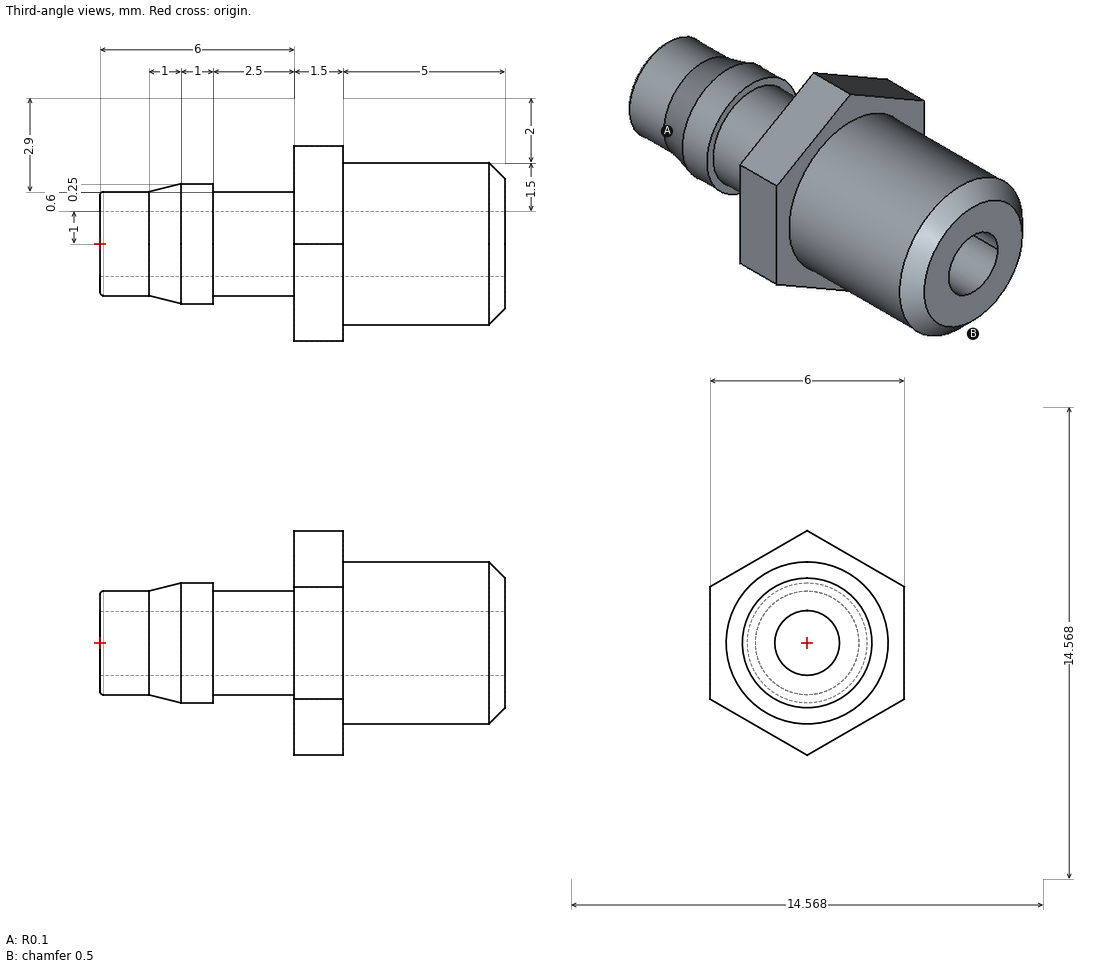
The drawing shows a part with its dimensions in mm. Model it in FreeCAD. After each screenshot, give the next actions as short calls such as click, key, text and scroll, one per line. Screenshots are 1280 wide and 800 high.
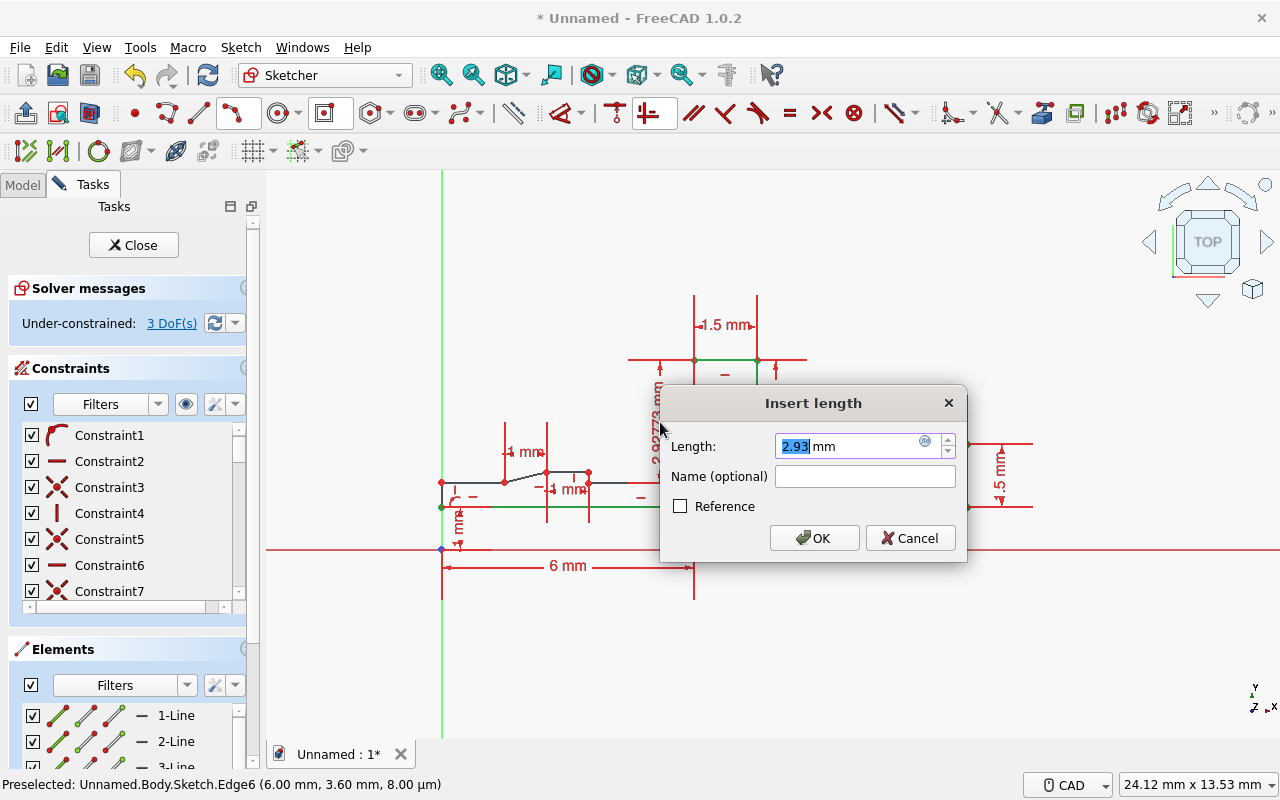
text(2.9)
key(Return)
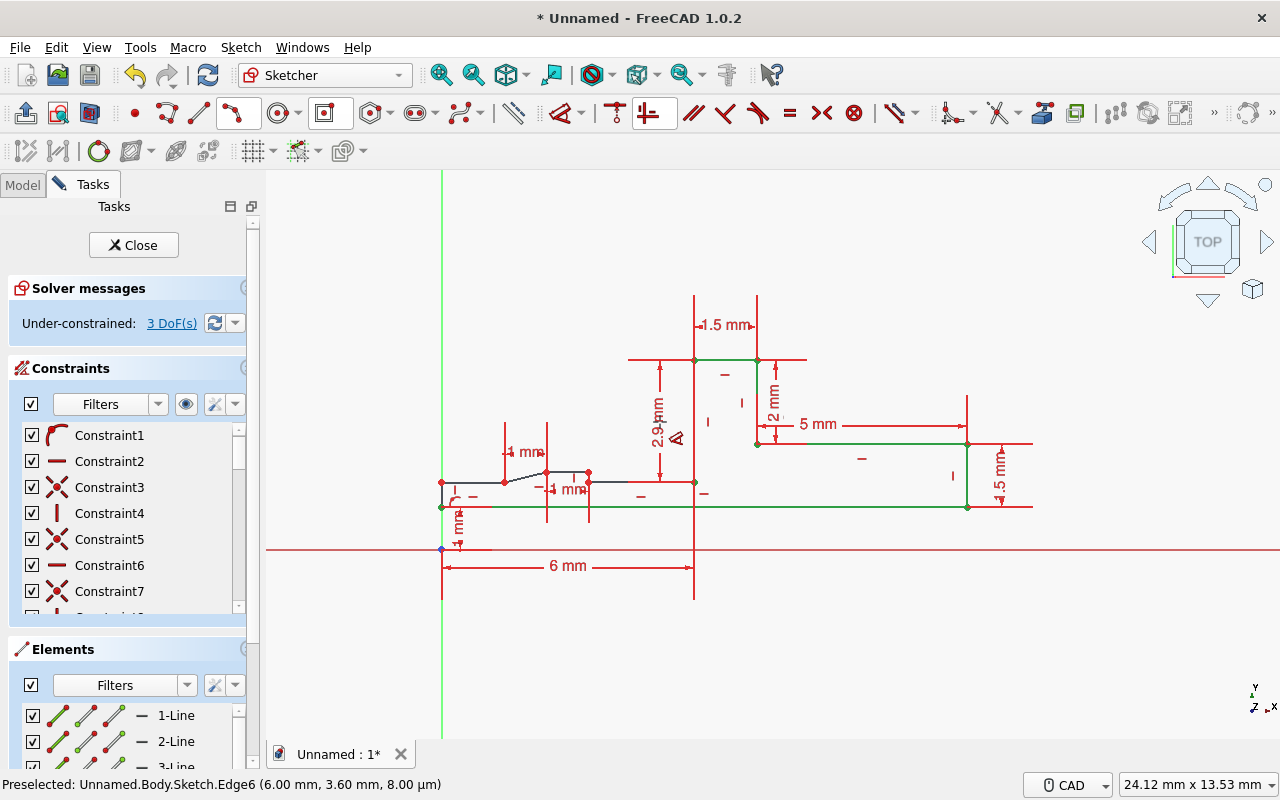
click(662, 482)
click(641, 448)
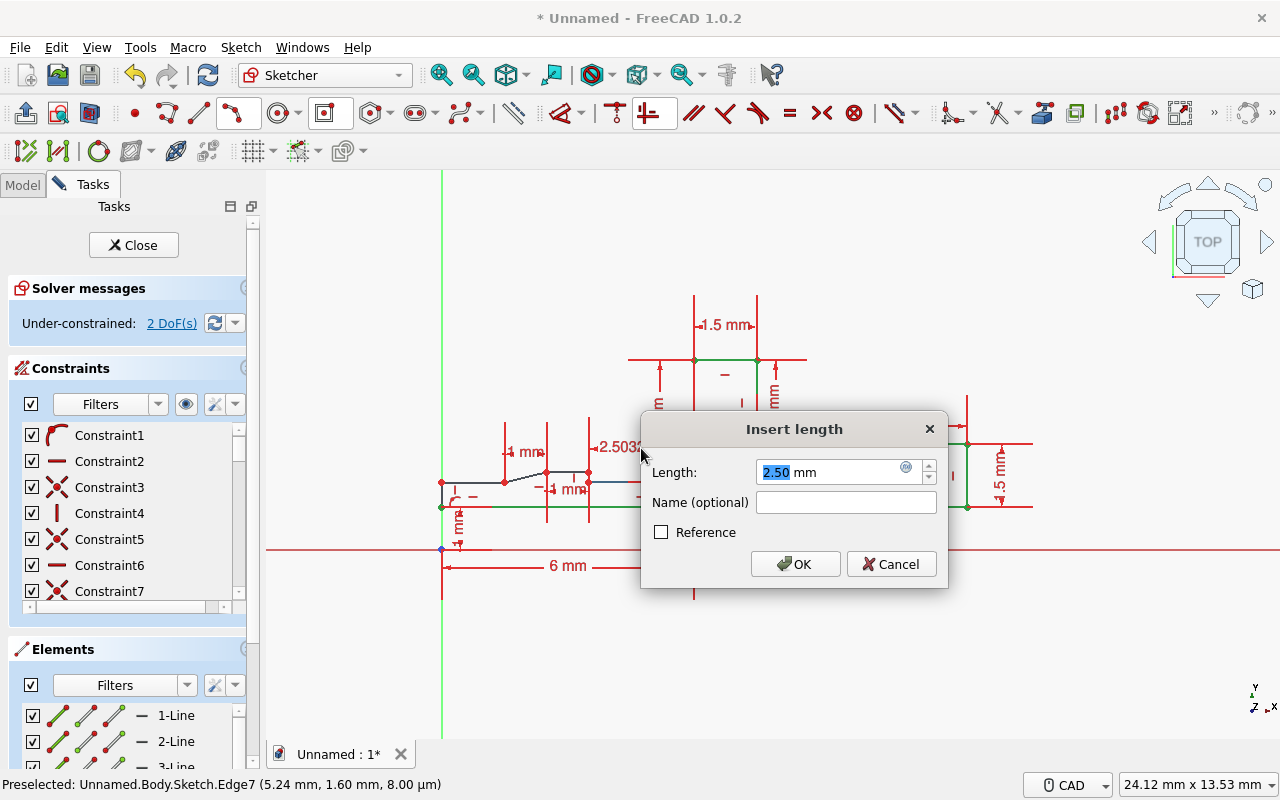
text(2.5)
key(Return)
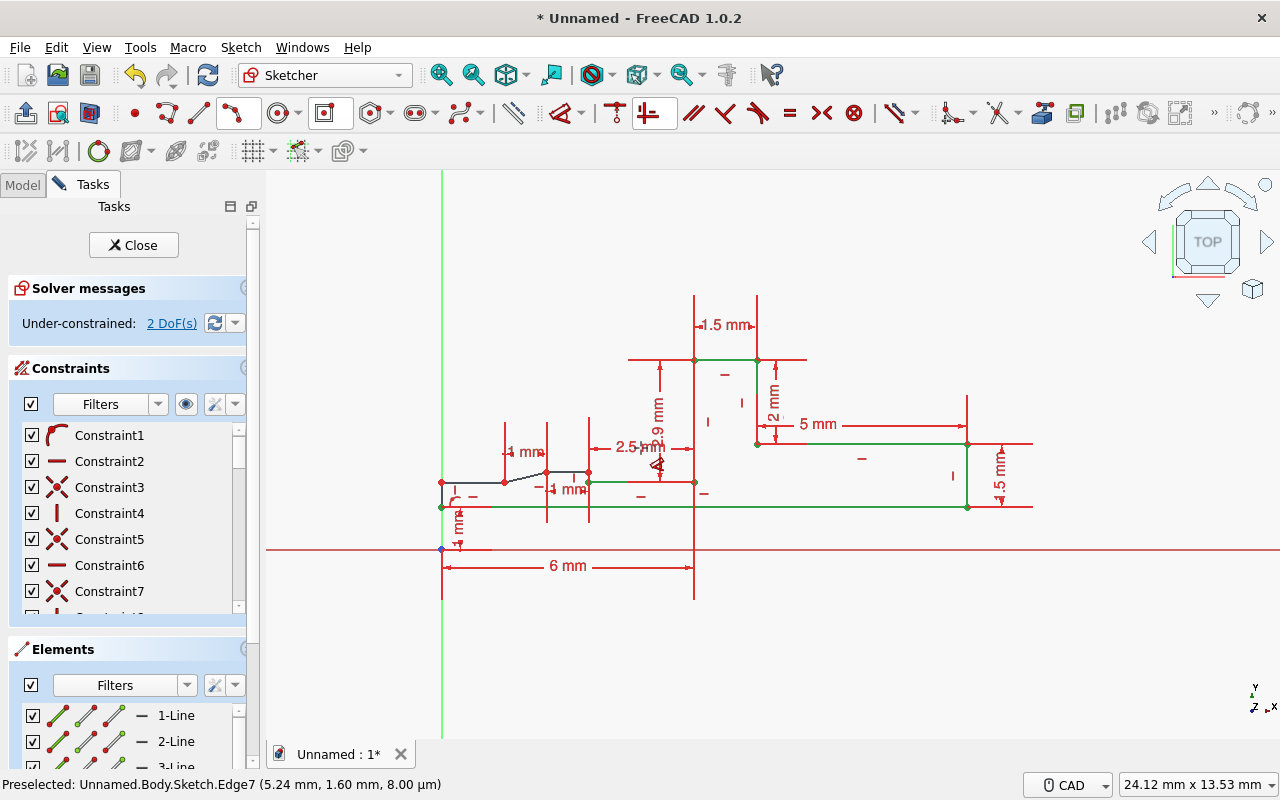
scroll(442, 493, up, 3)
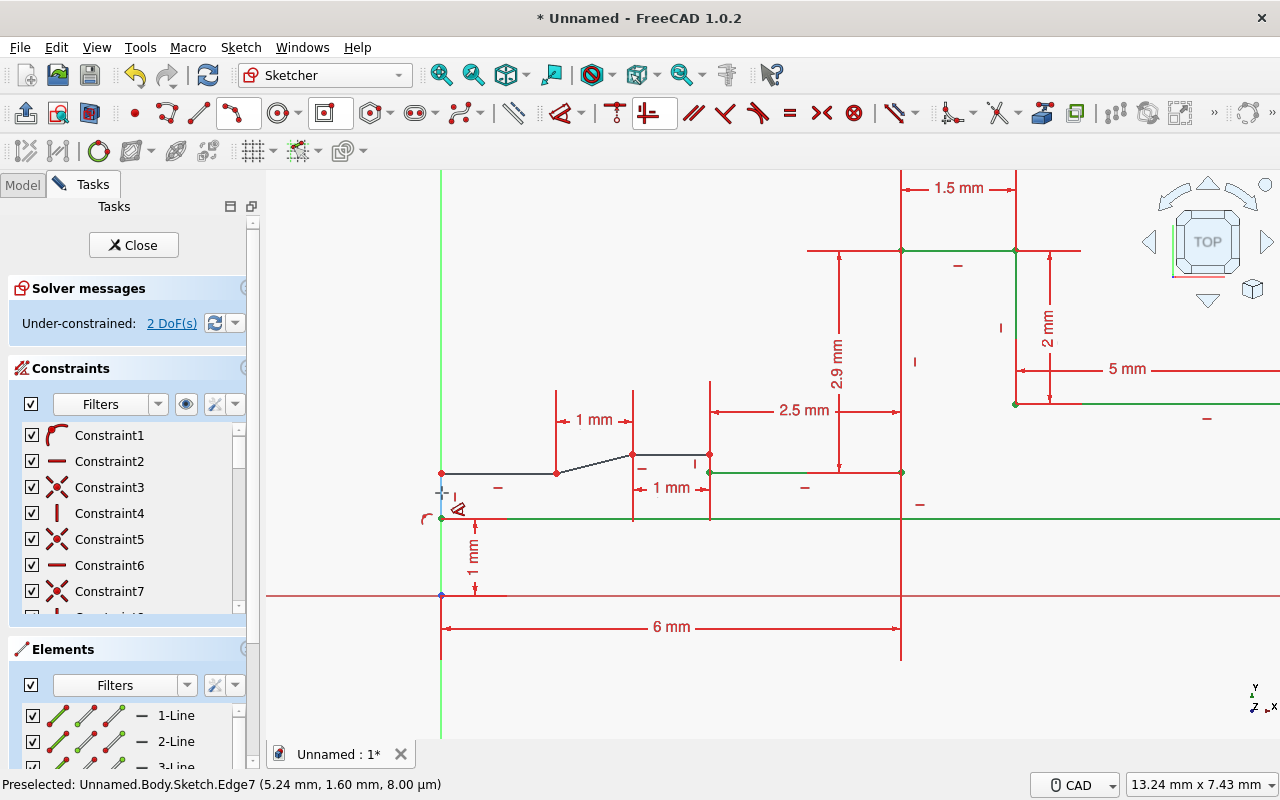
click(441, 492)
click(407, 496)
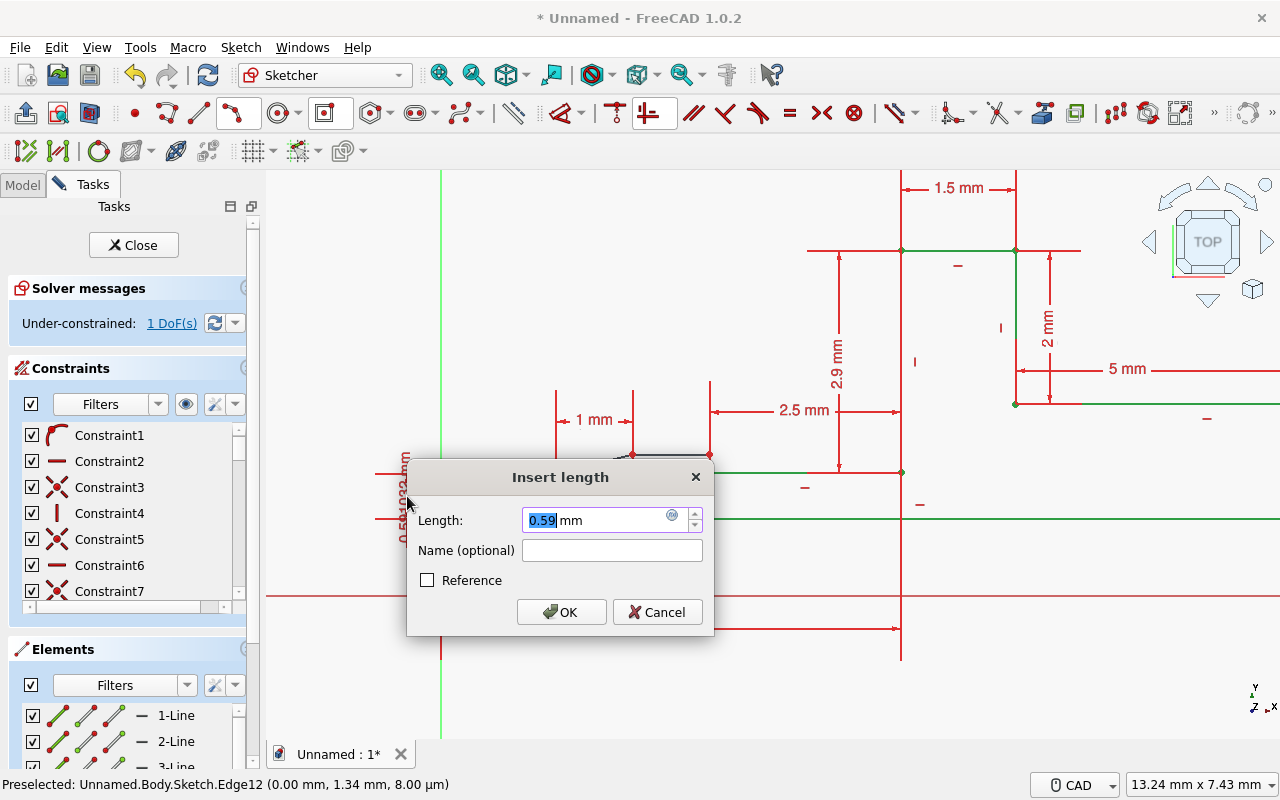
text(0.6)
key(Return)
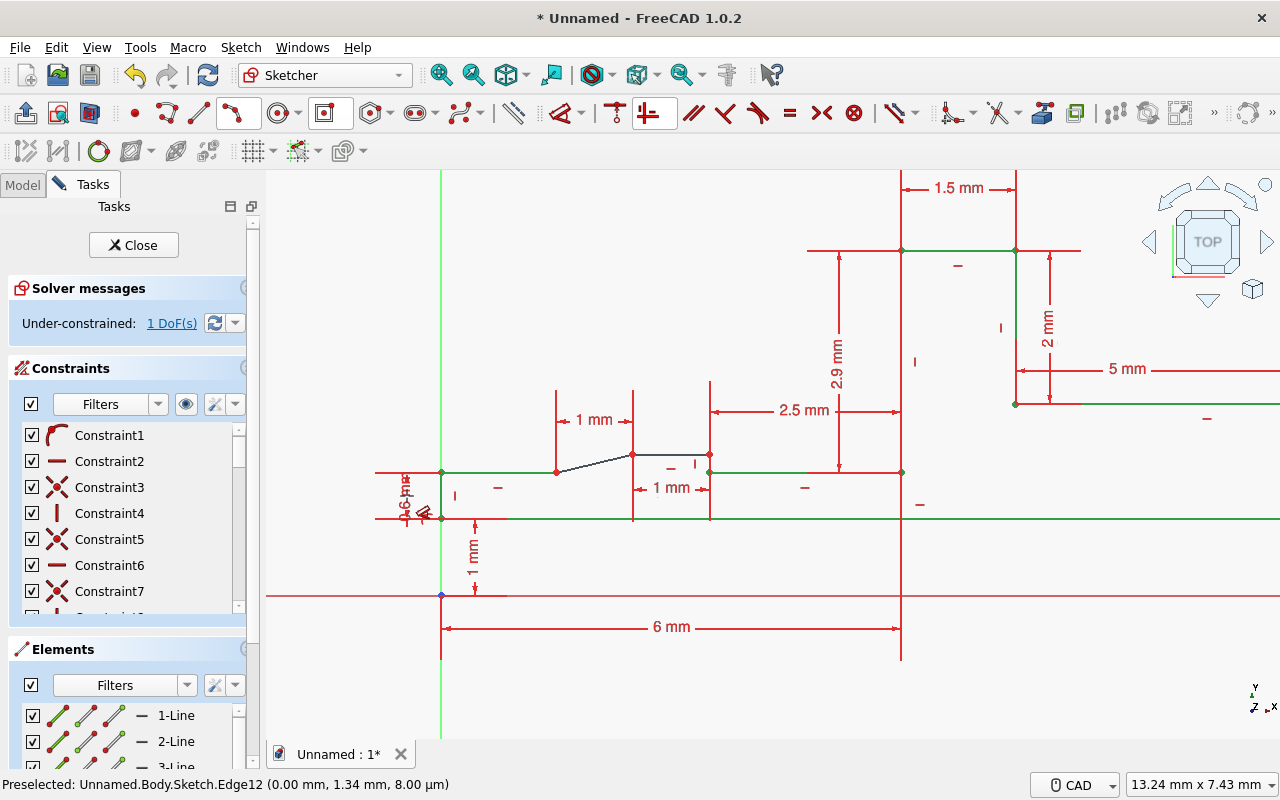
scroll(710, 464, up, 4)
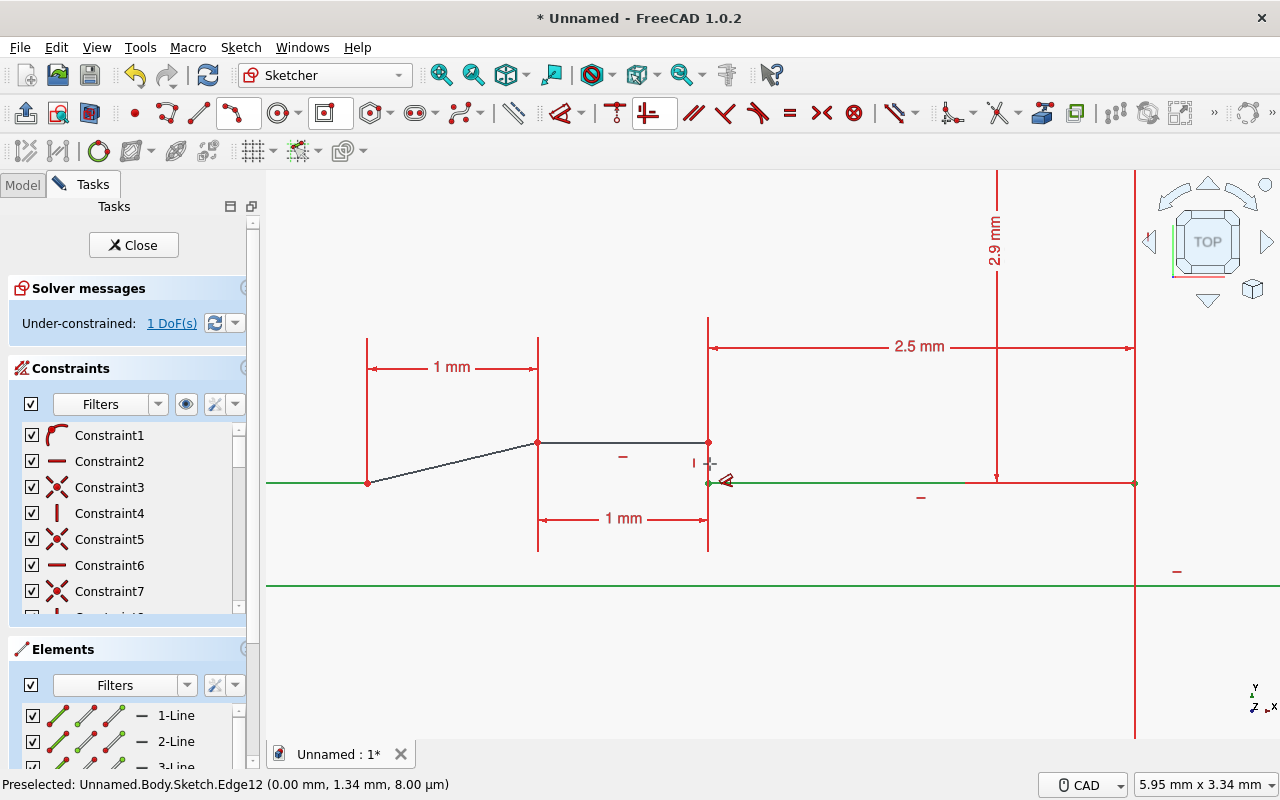
click(708, 463)
click(674, 463)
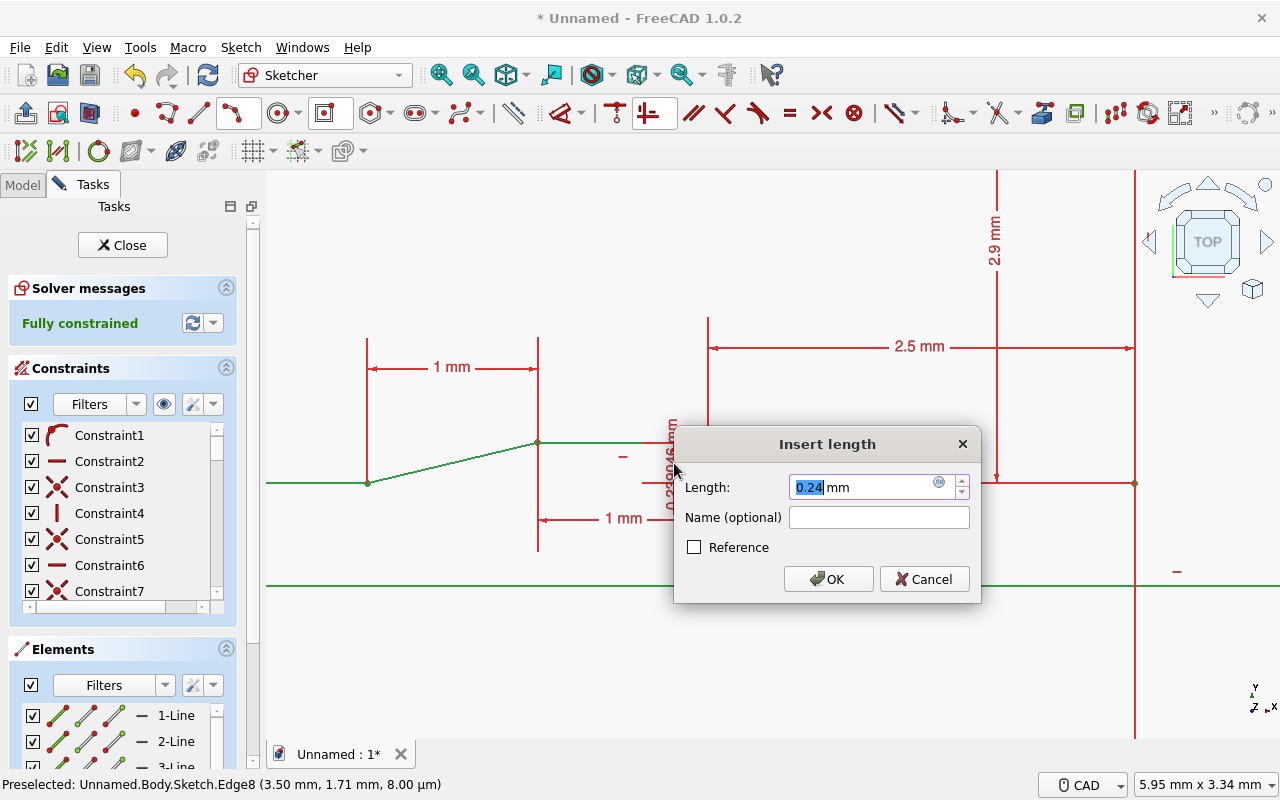
text(0.25)
key(Return)
key(Escape)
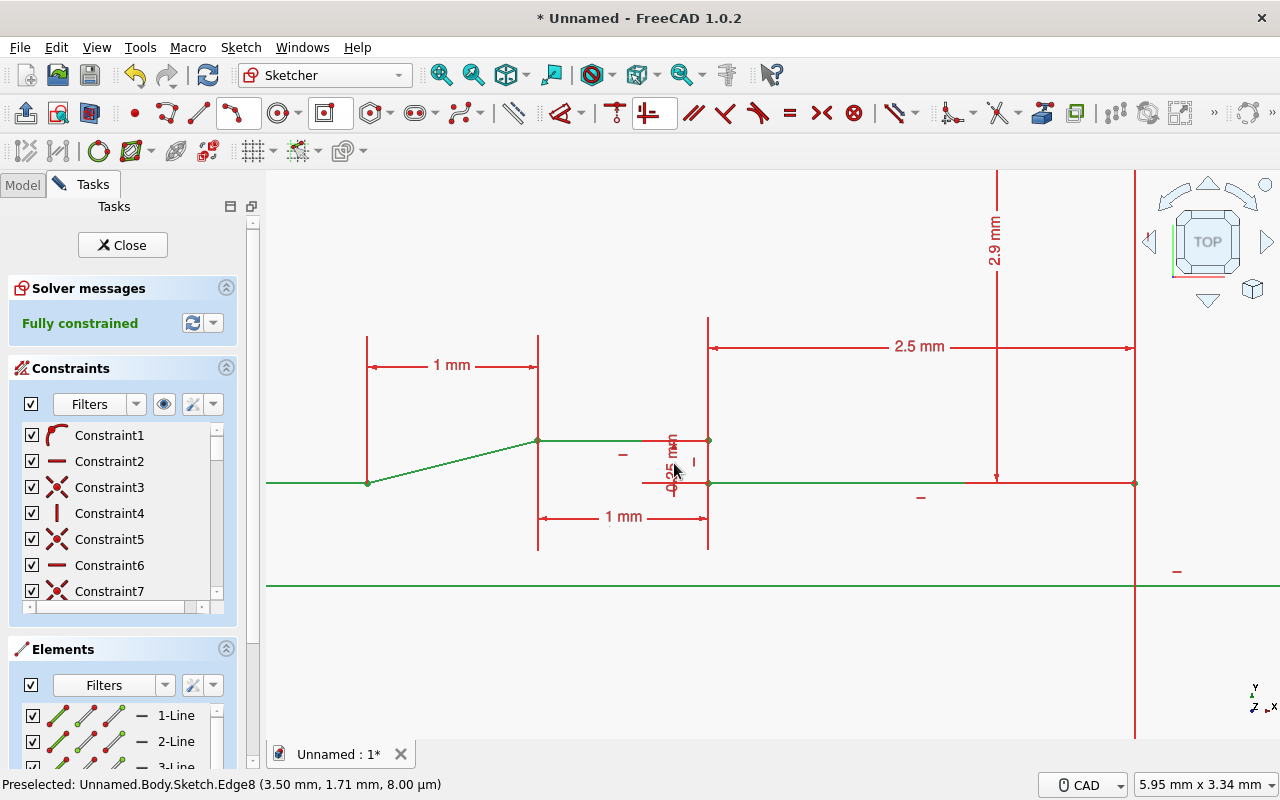
click(123, 245)